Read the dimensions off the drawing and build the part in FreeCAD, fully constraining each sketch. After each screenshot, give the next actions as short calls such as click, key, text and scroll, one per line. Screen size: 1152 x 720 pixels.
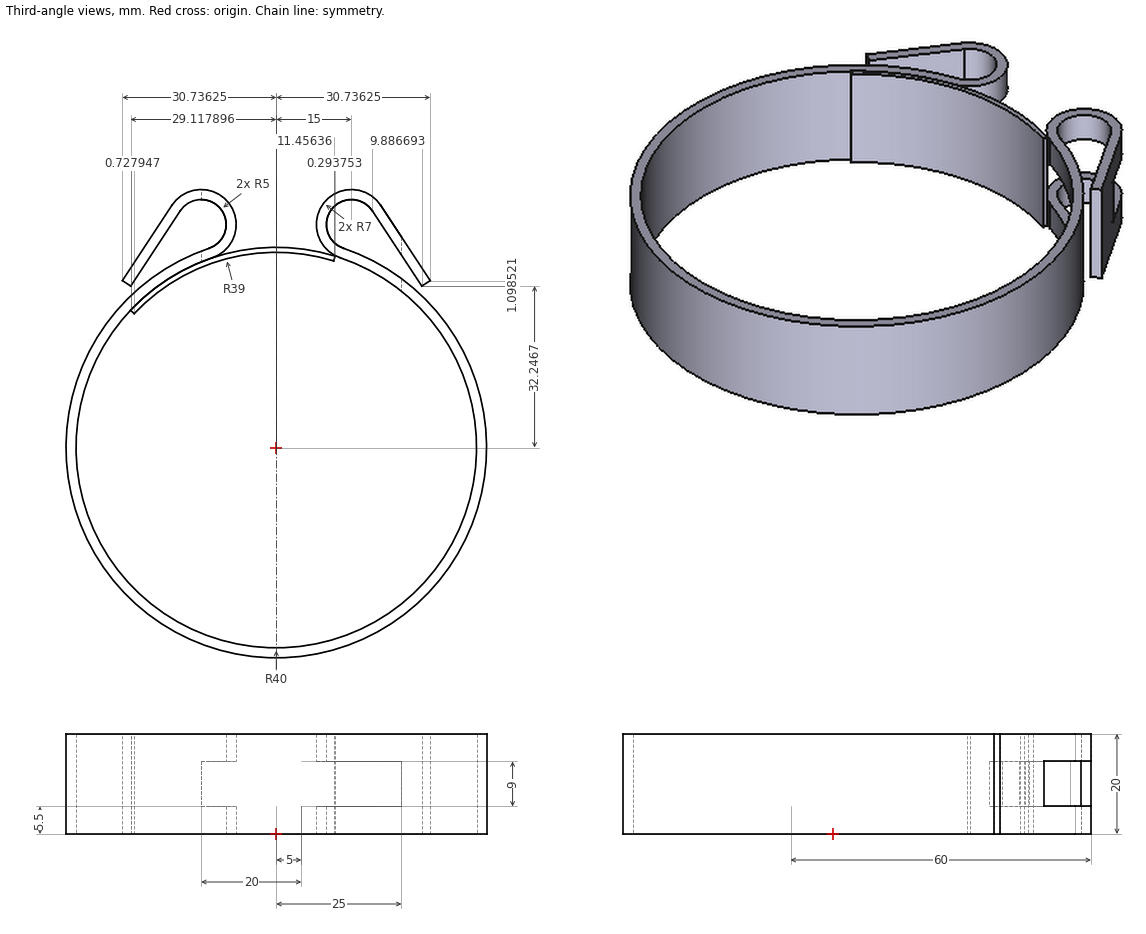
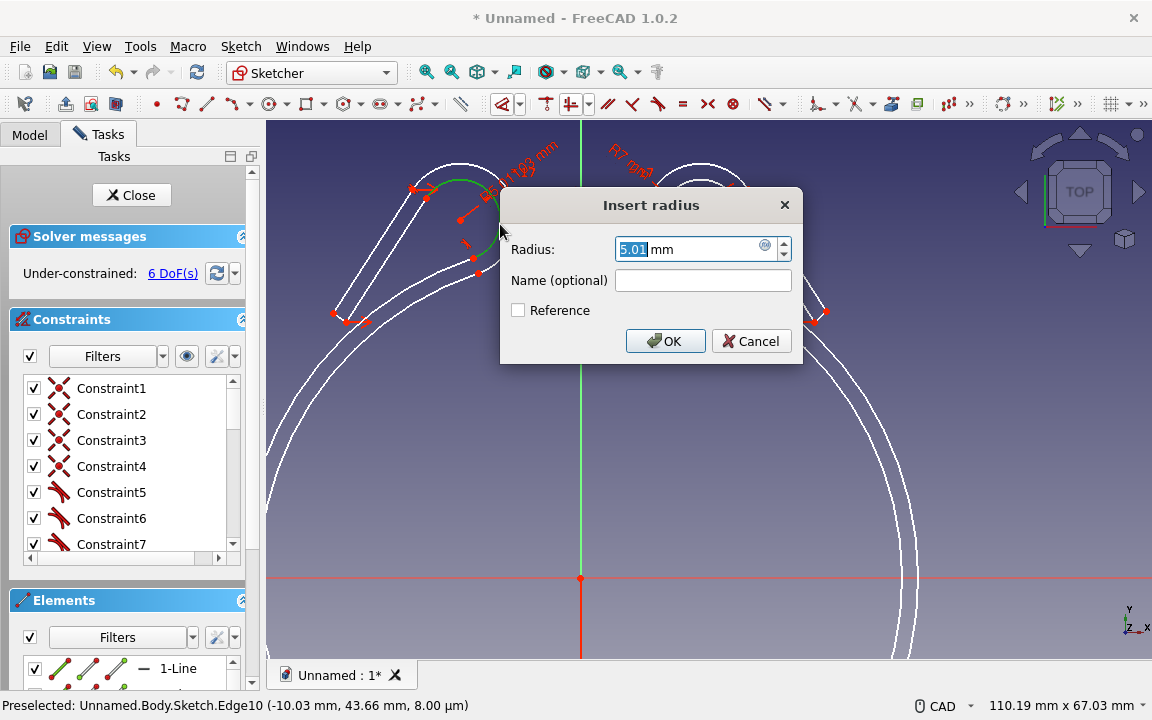
text(5)
key(Return)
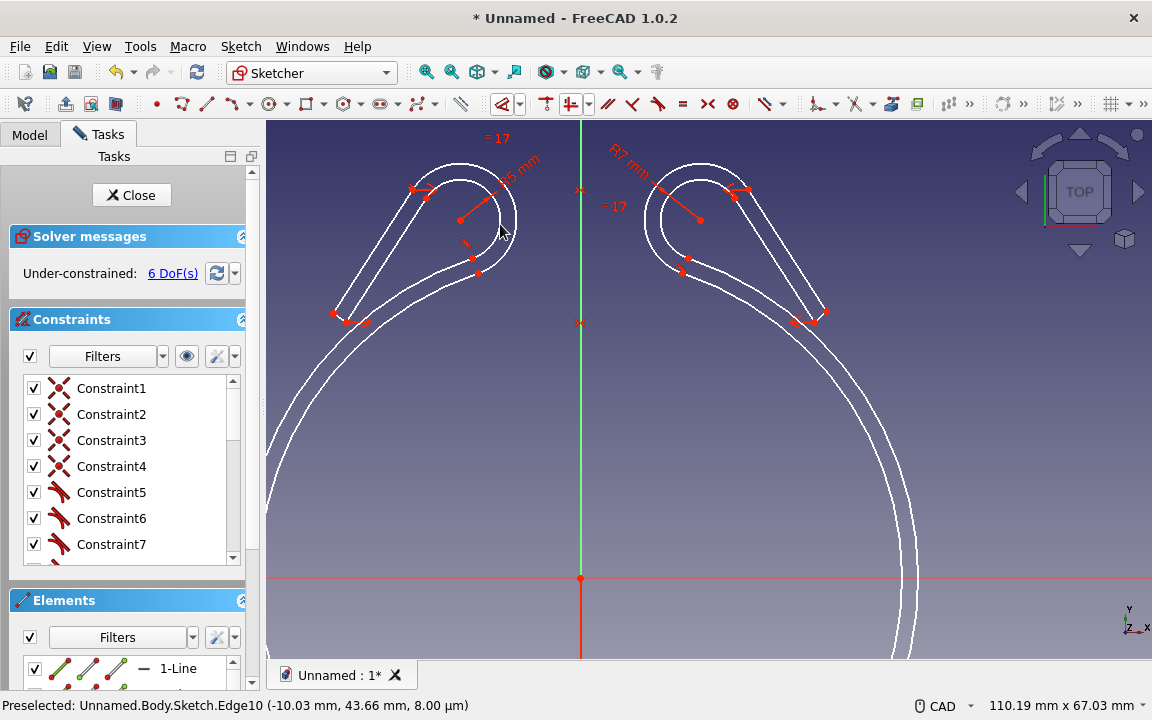
click(701, 220)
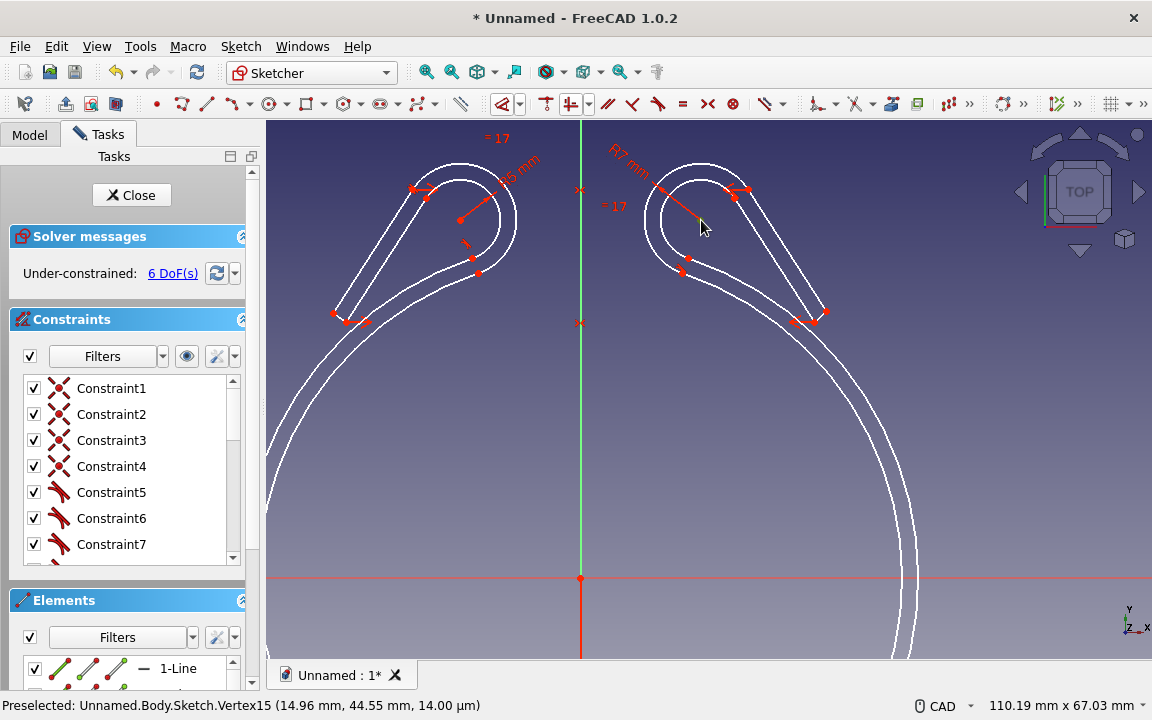
key(l)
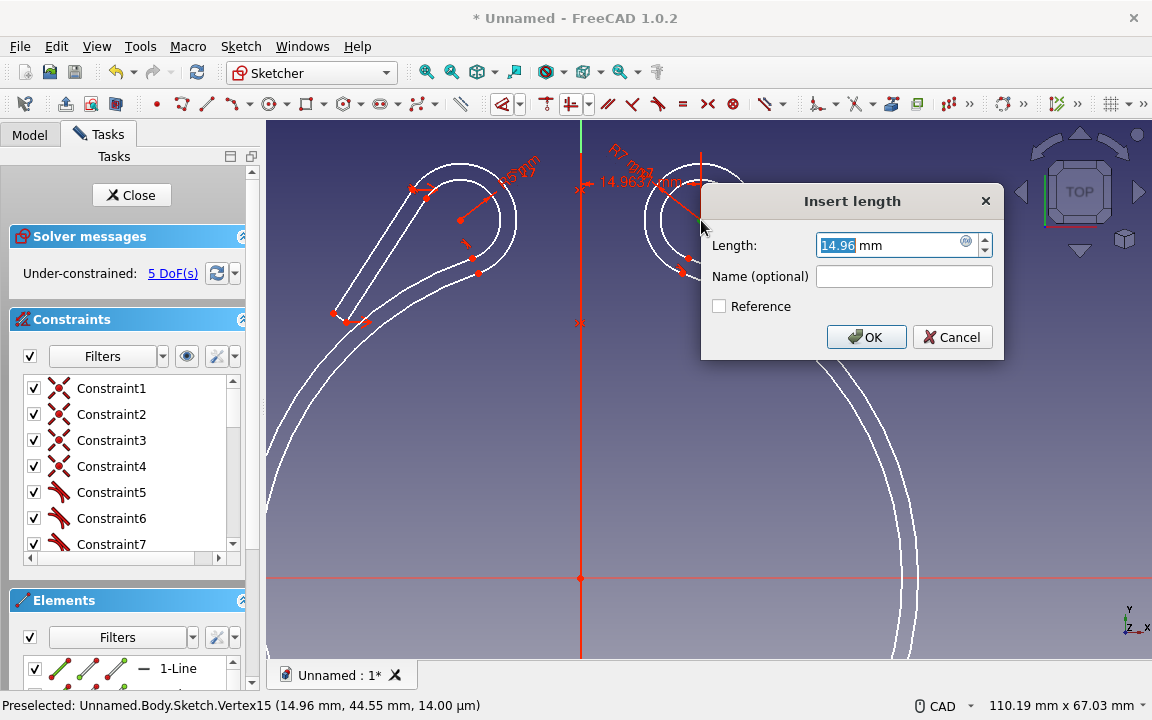
text(15)
key(Return)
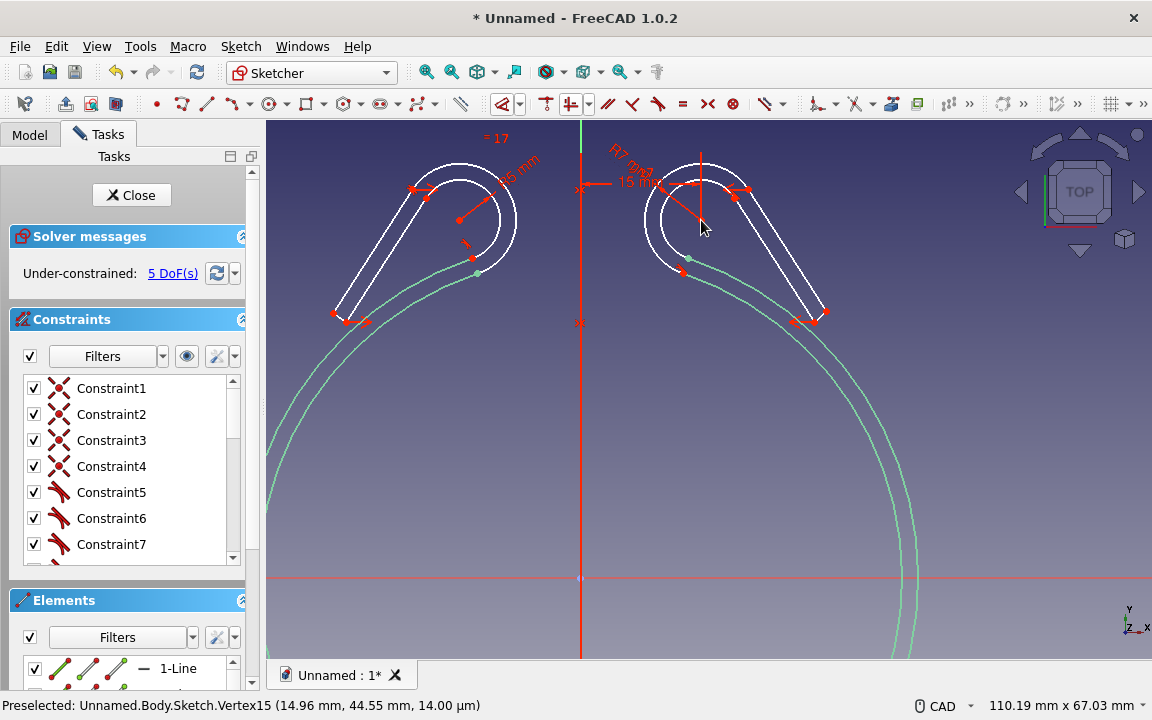
click(815, 322)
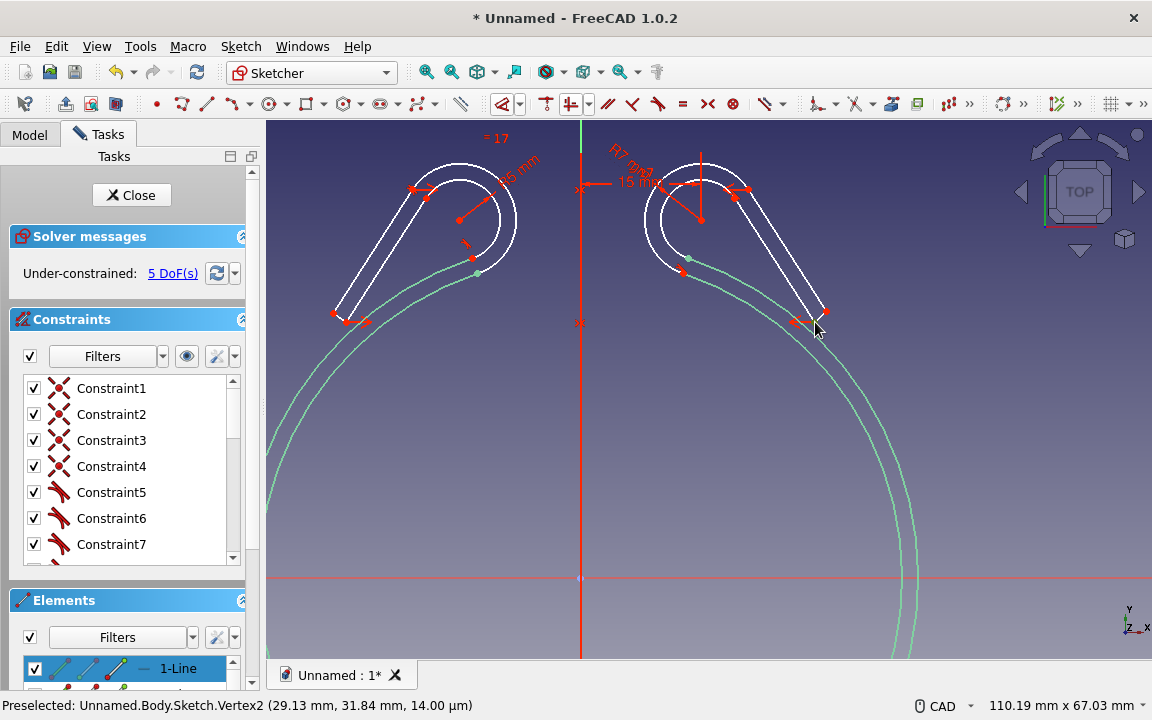
click(520, 104)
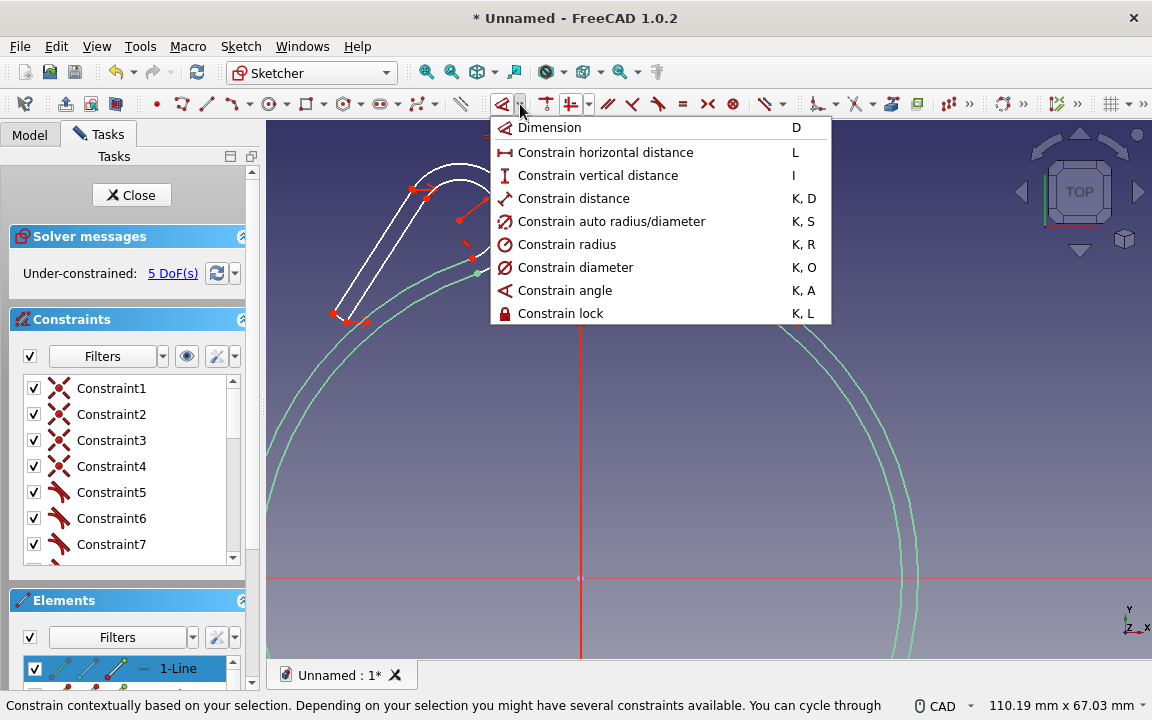
click(661, 176)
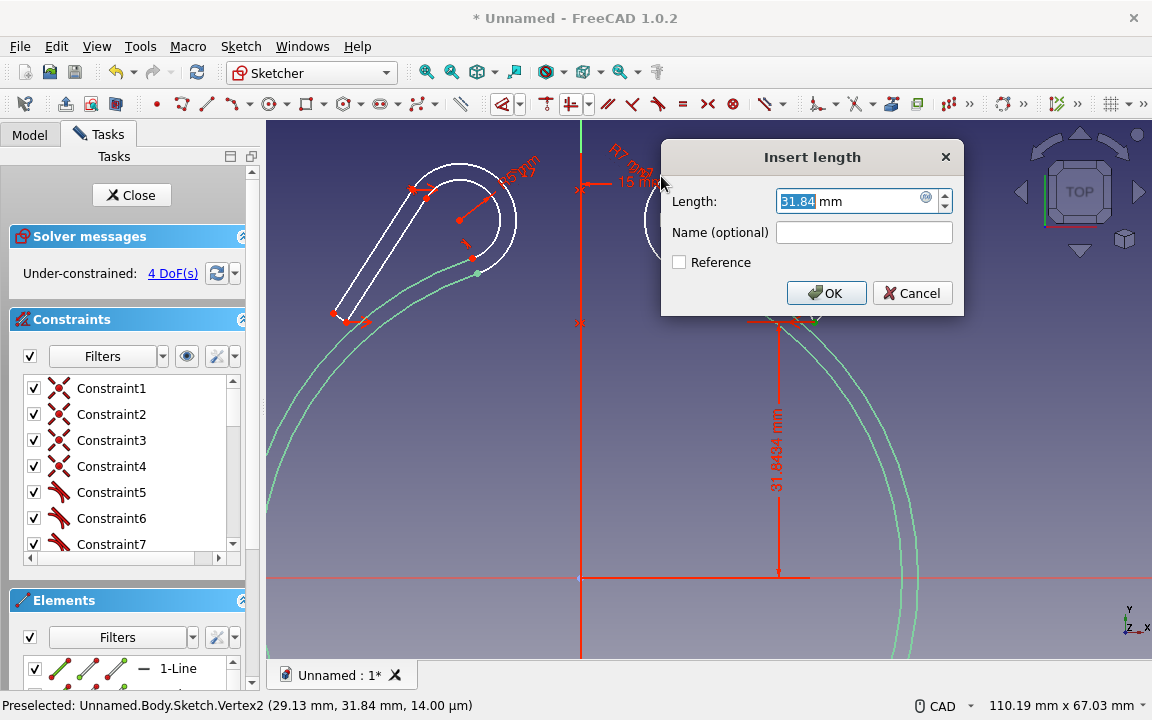
text(32.2467)
key(Return)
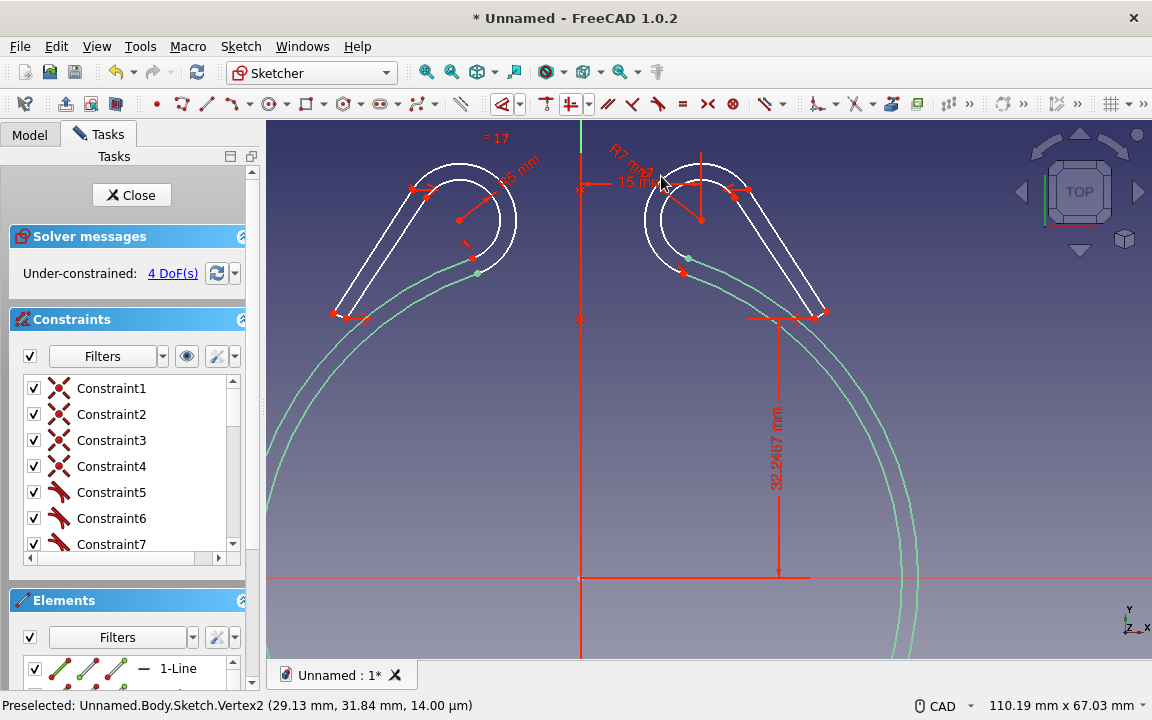
click(826, 311)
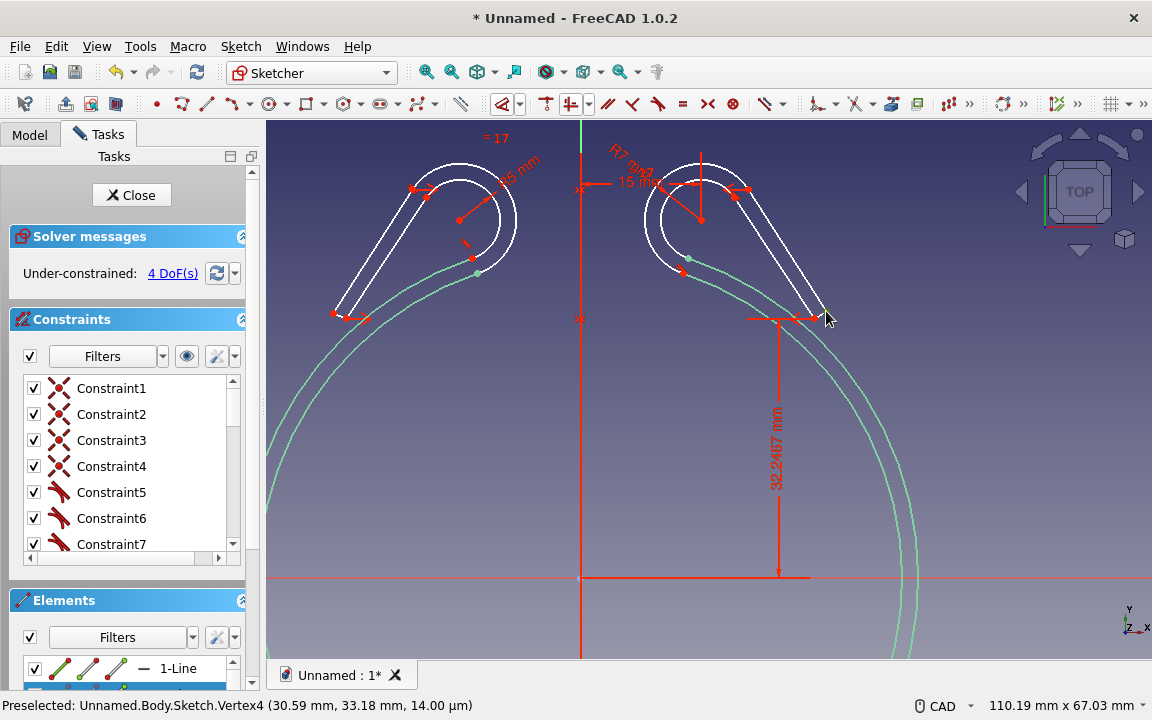
key(l)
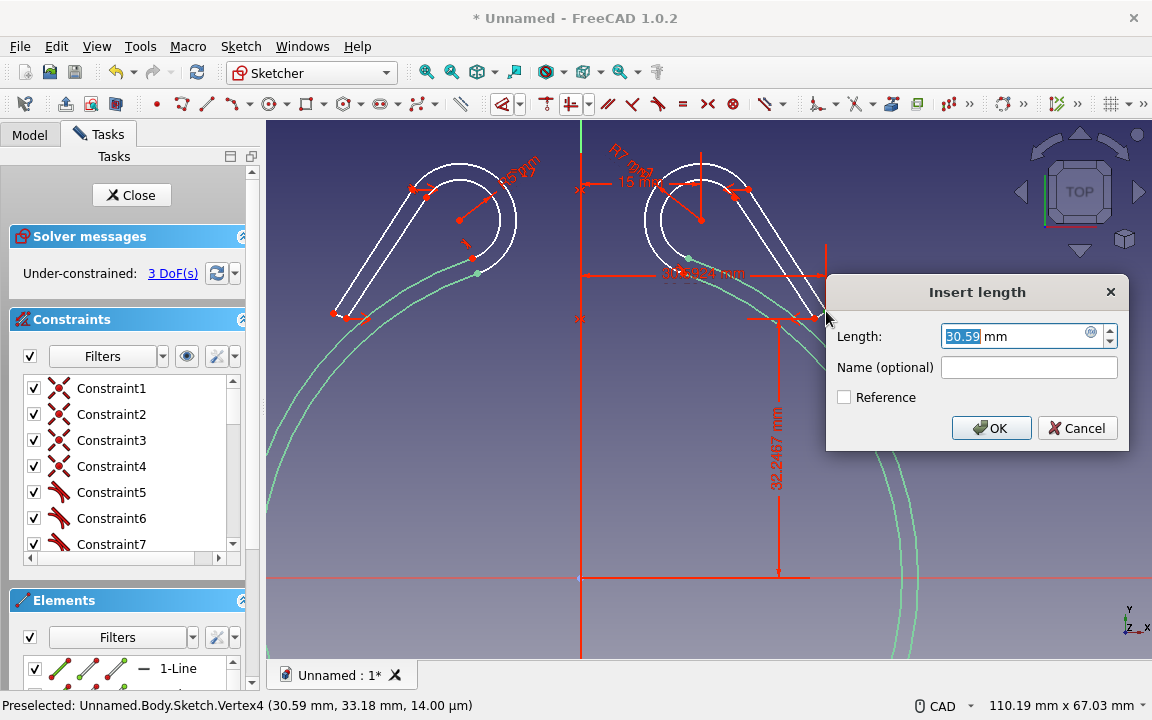
text(30.73625)
key(Return)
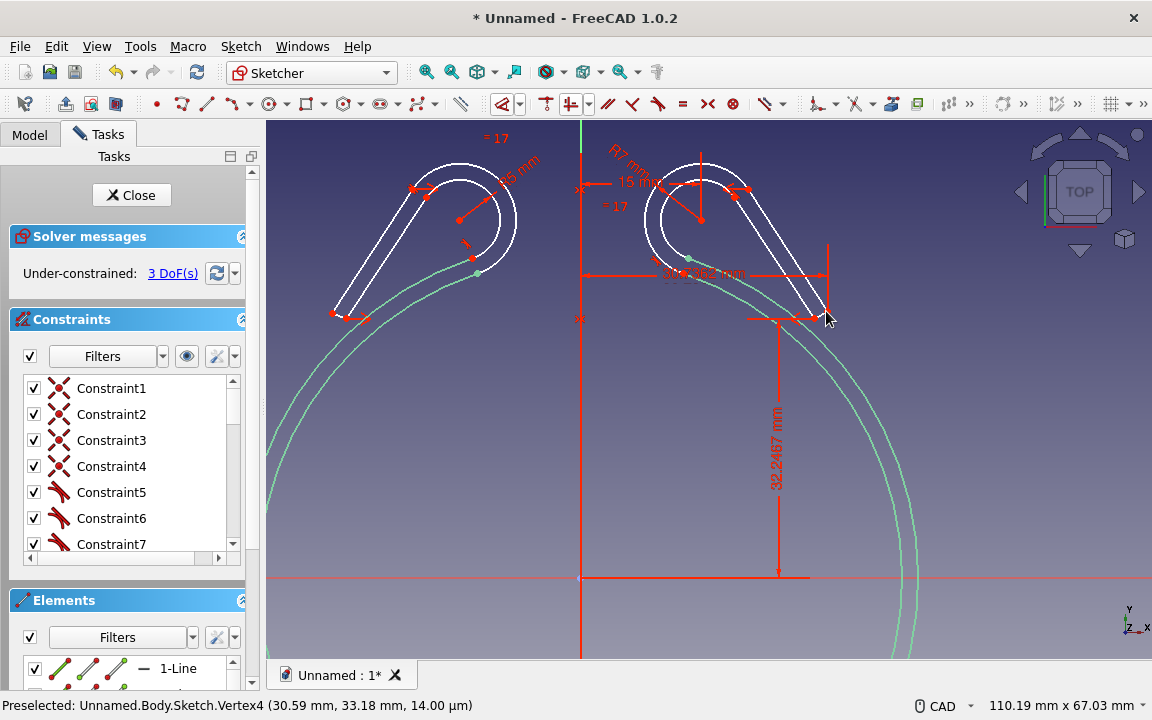
click(332, 313)